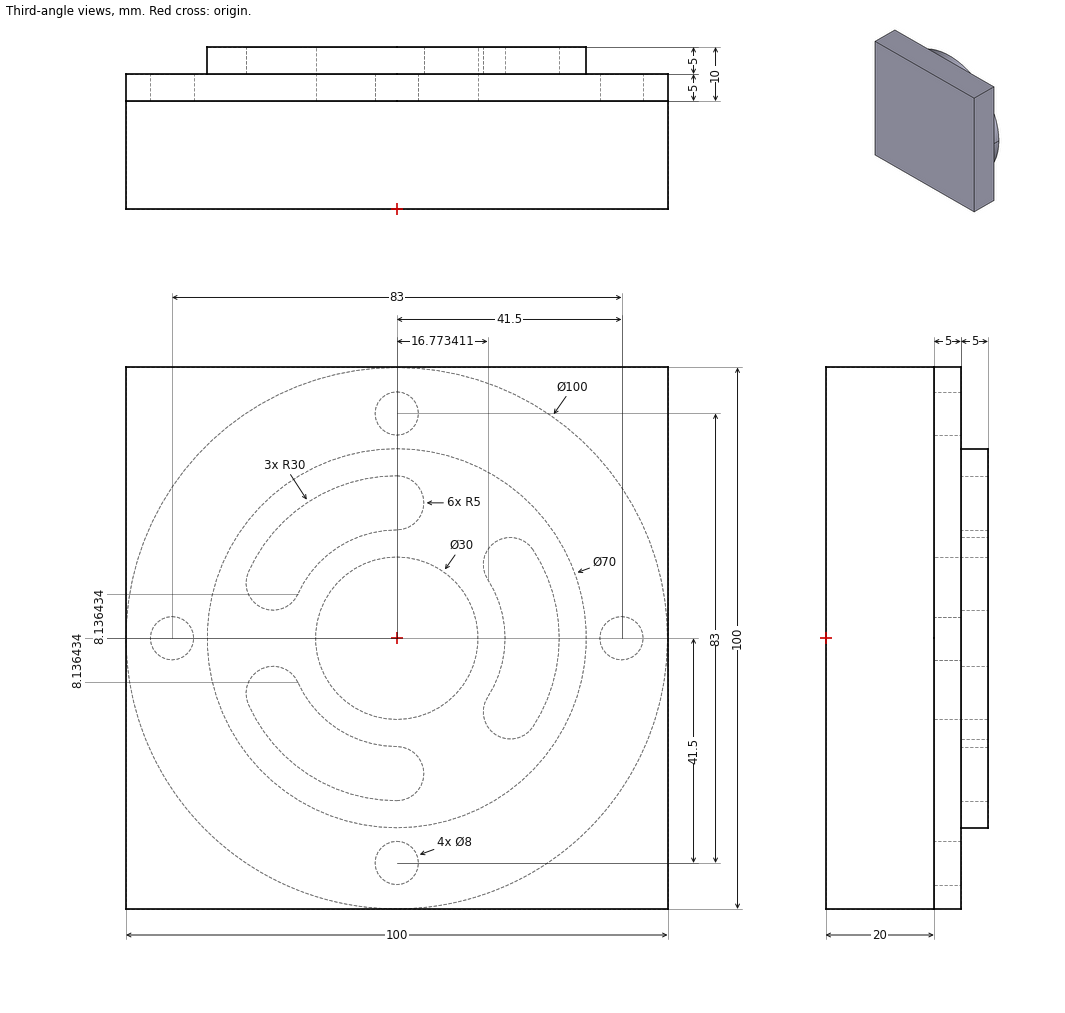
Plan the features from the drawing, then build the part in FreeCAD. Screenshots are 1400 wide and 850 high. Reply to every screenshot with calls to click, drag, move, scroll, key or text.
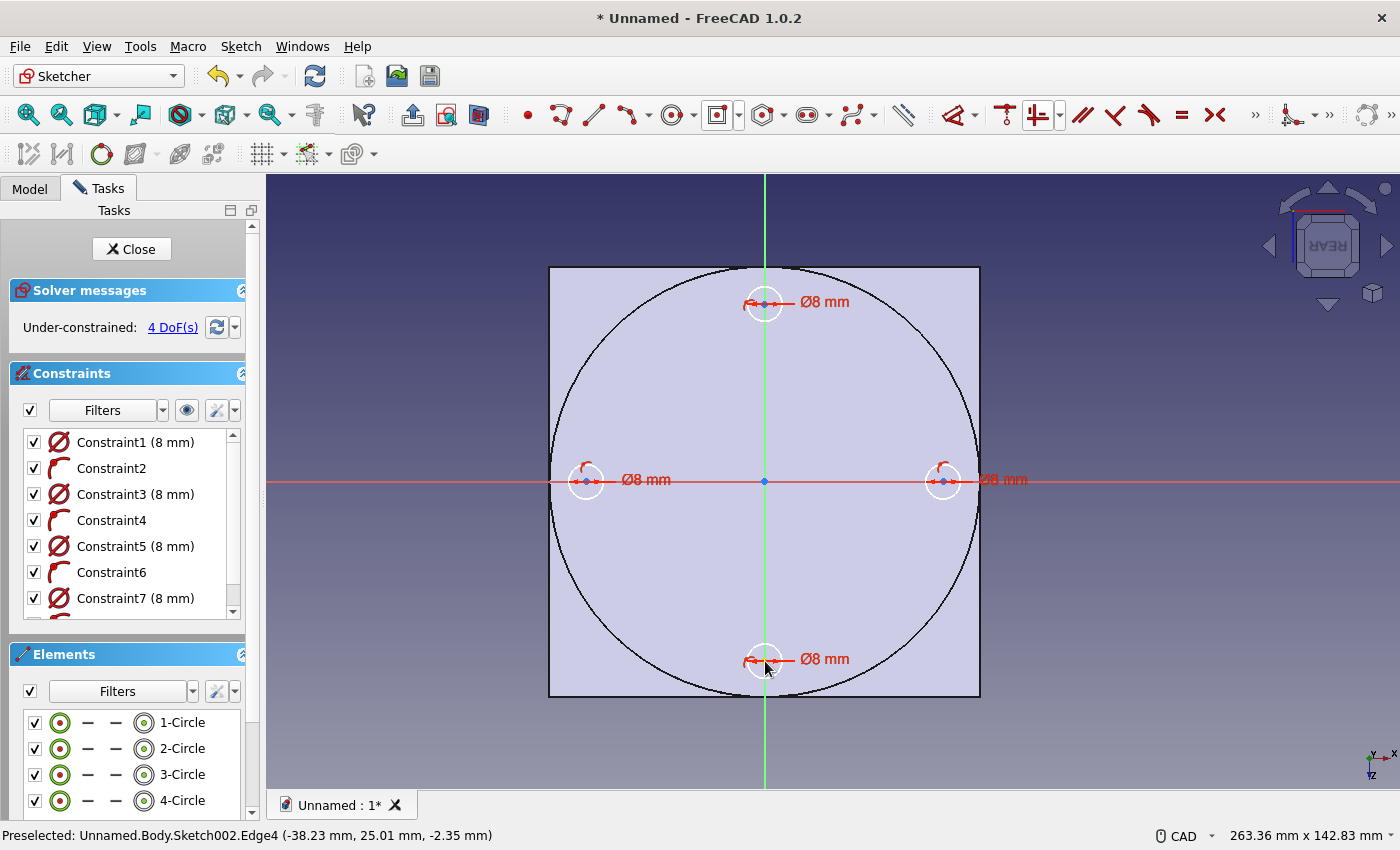
click(765, 304)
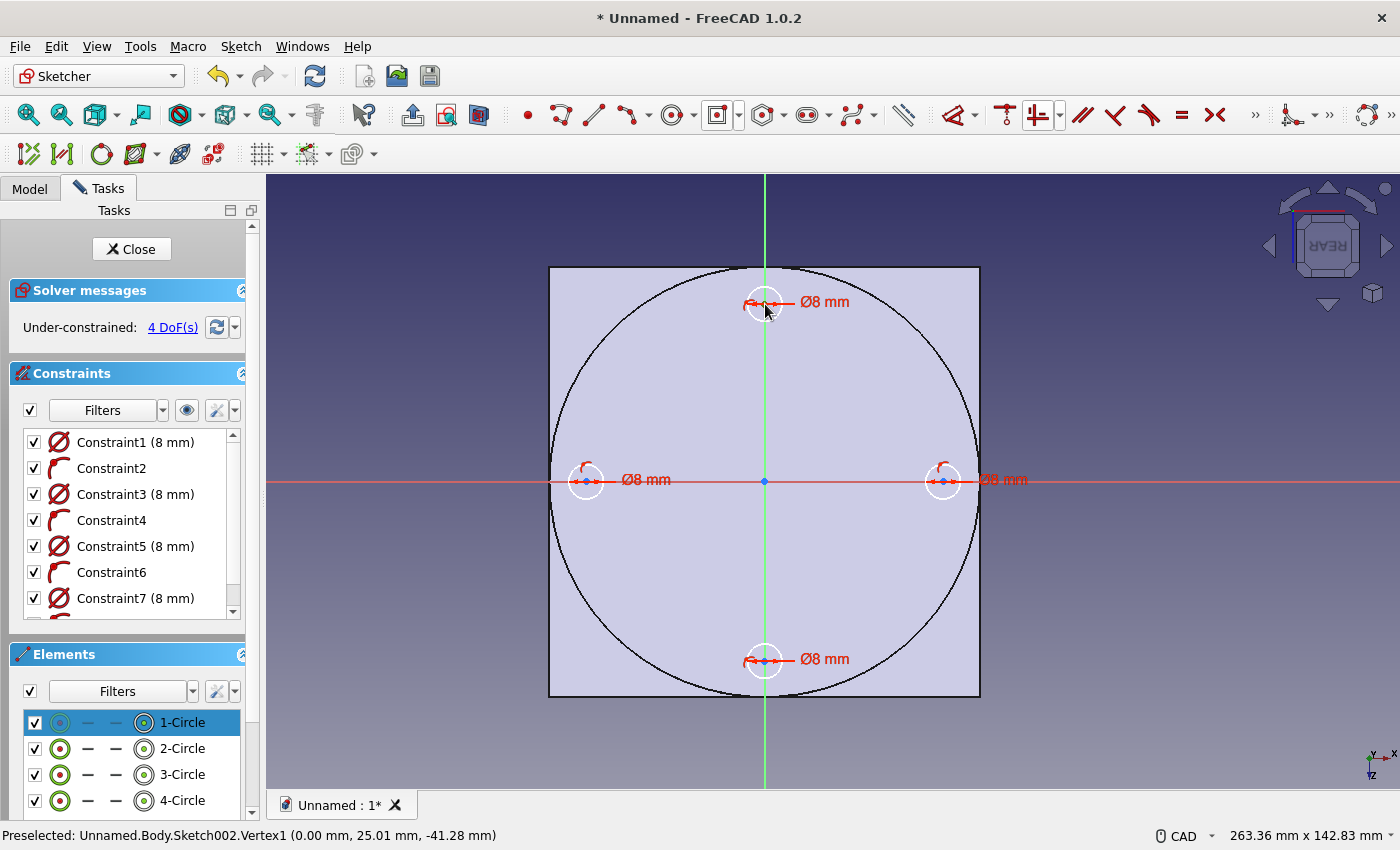
click(765, 661)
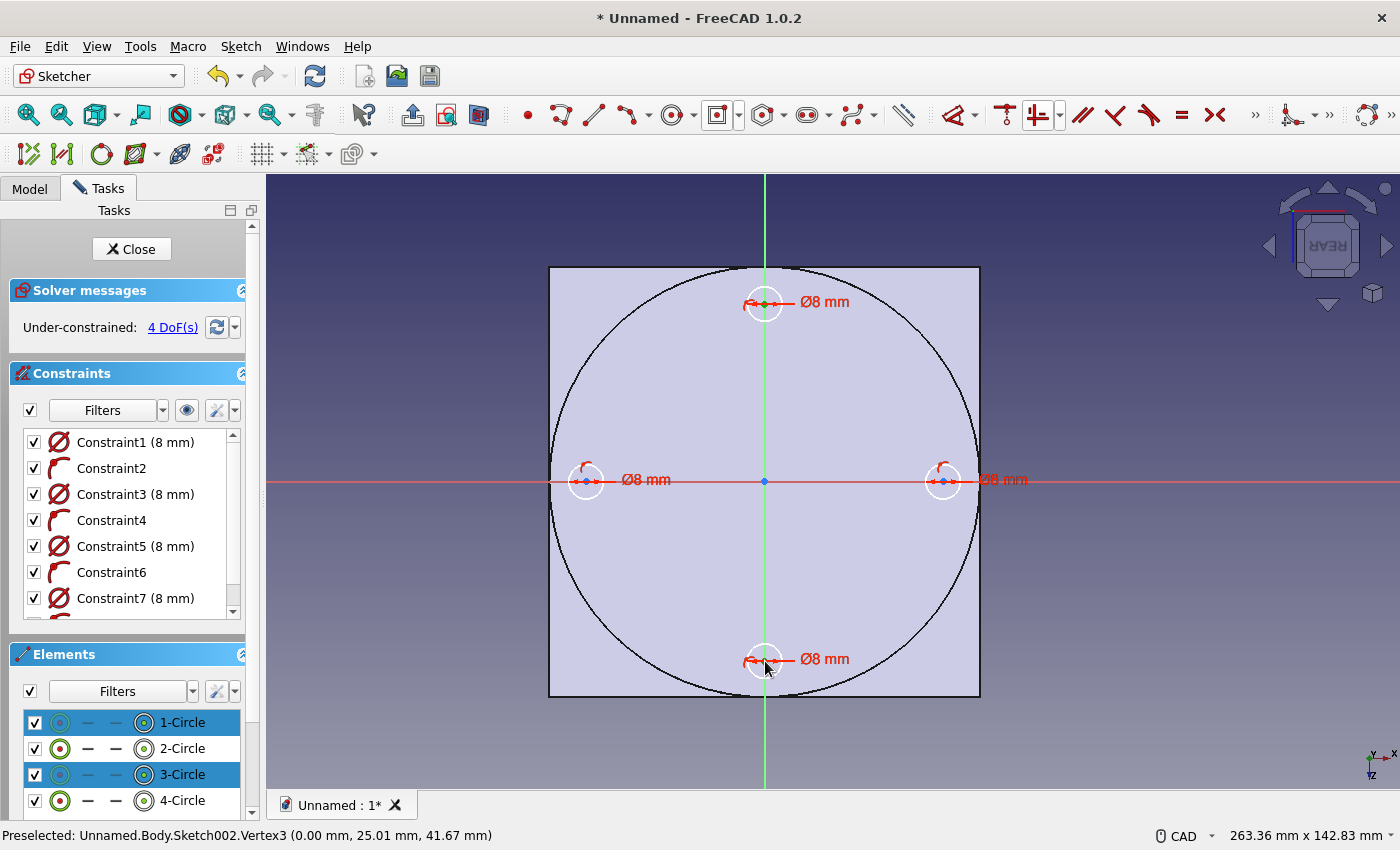
click(974, 116)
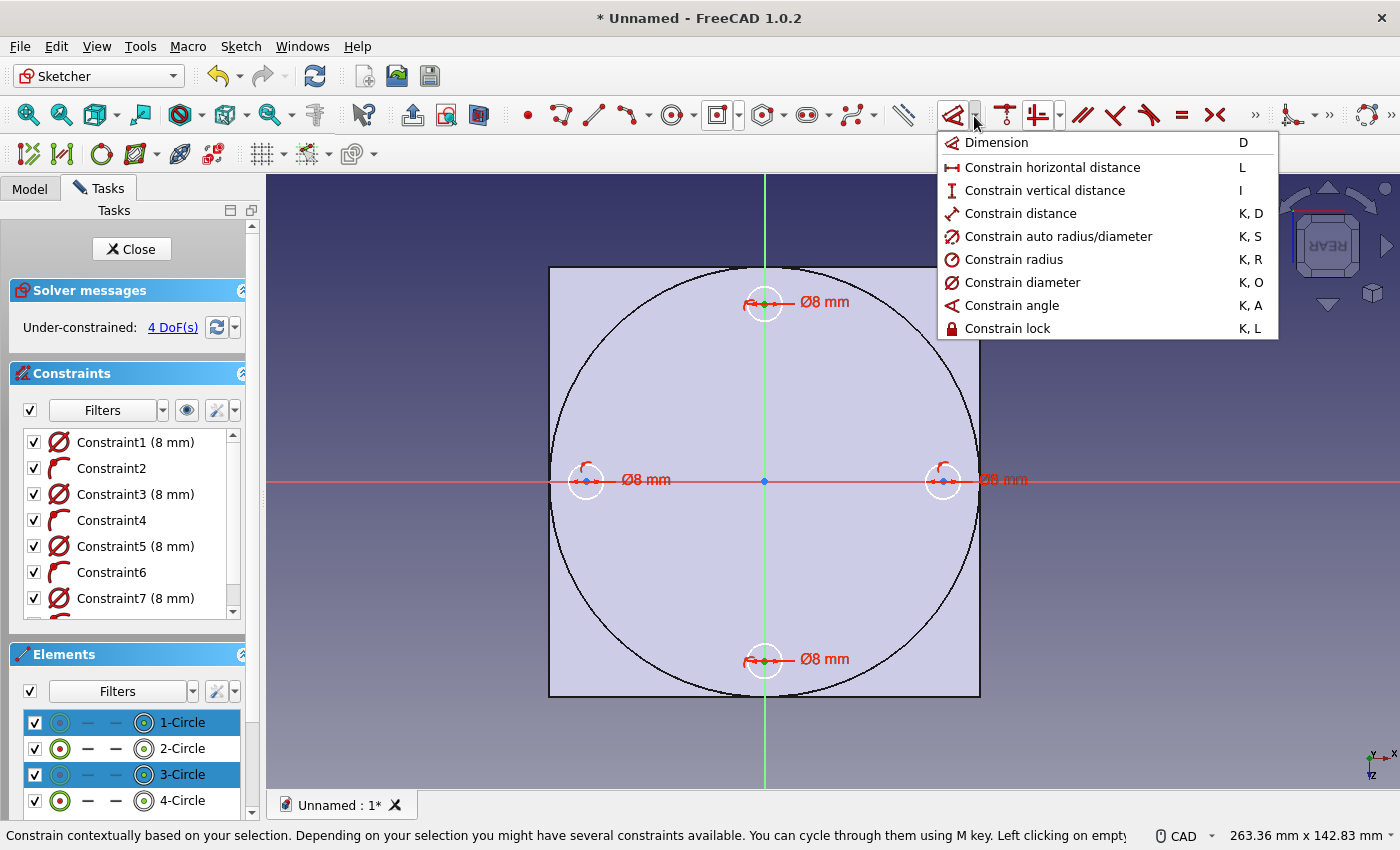
click(1108, 190)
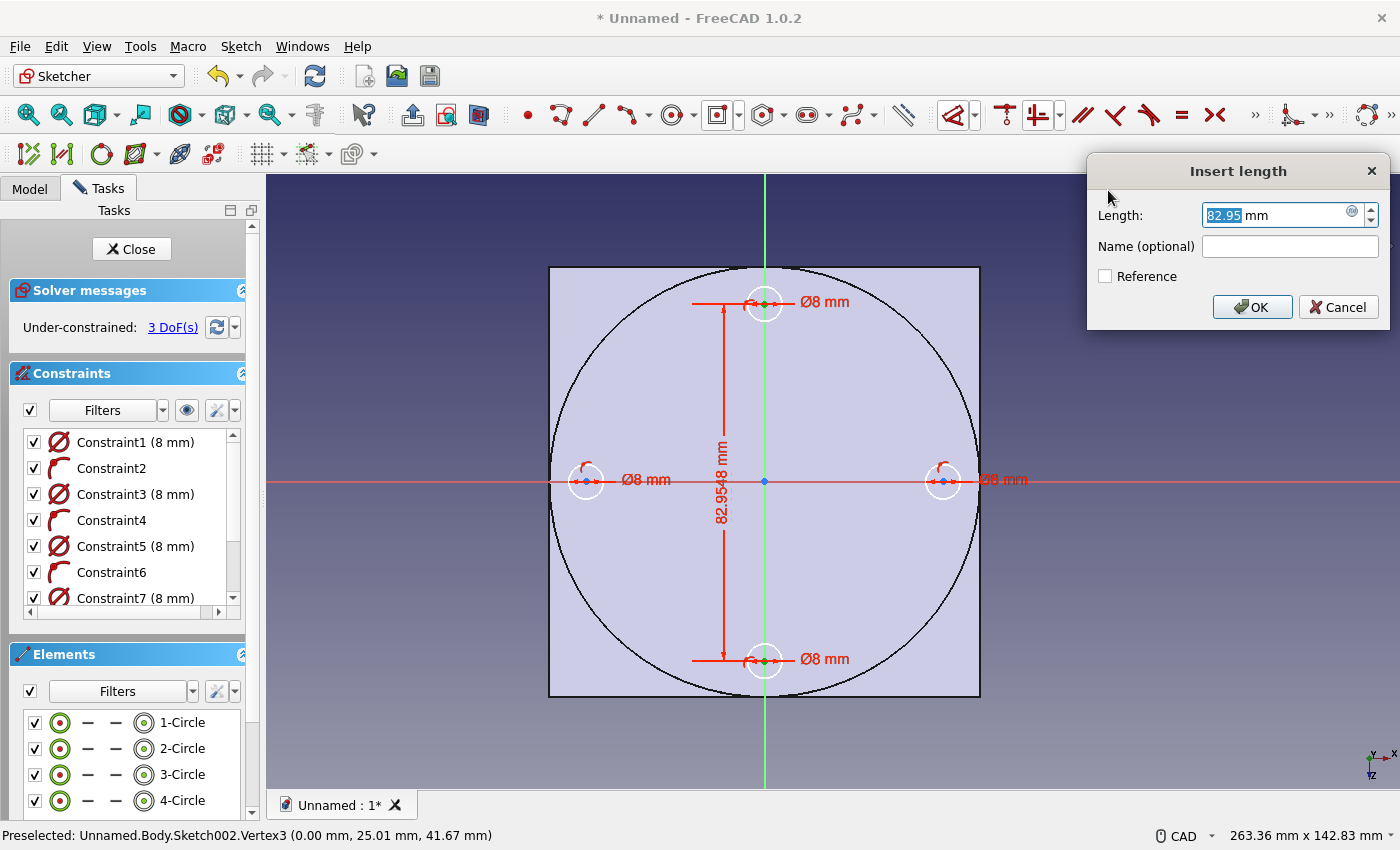
text(83)
key(Return)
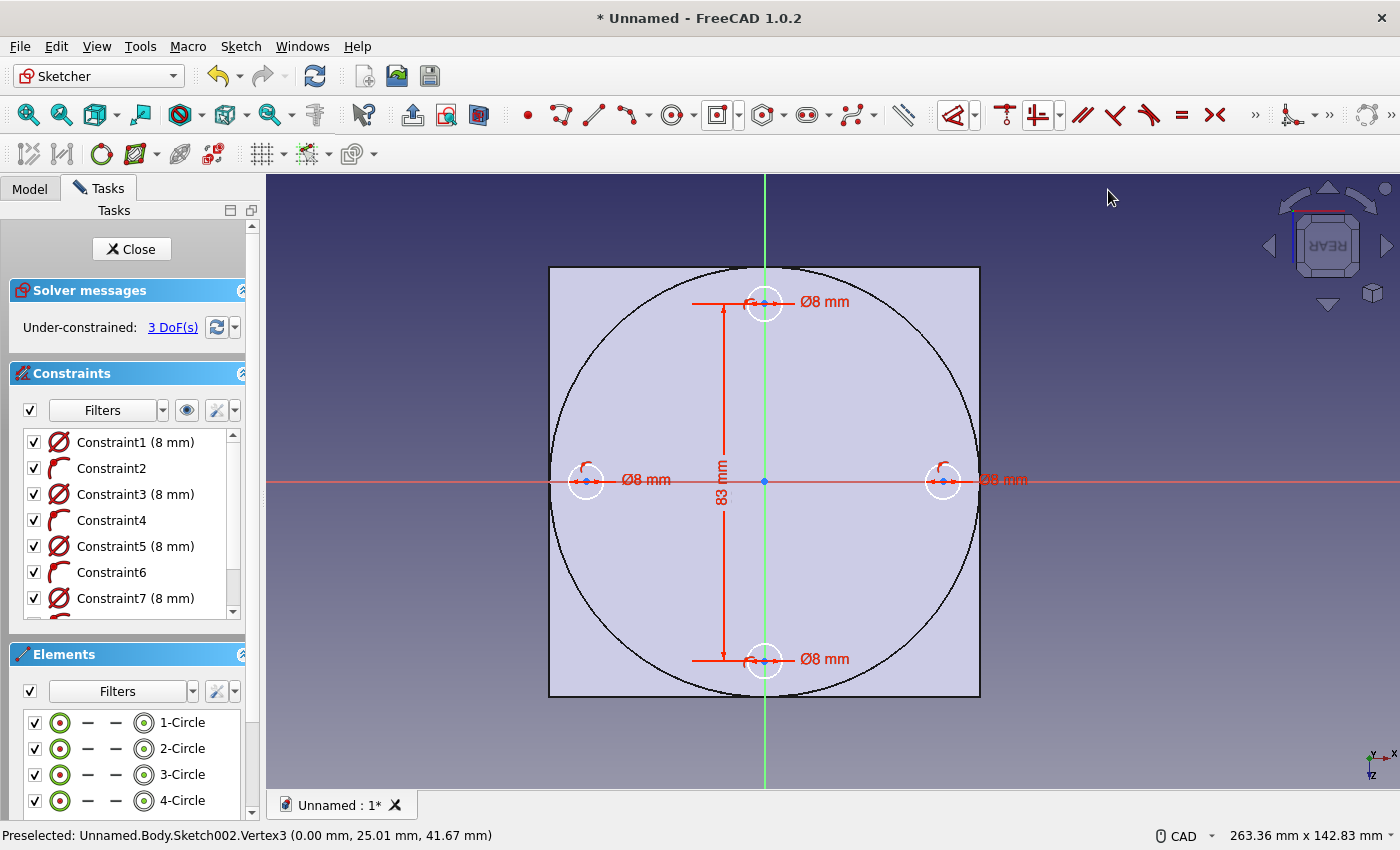
click(943, 482)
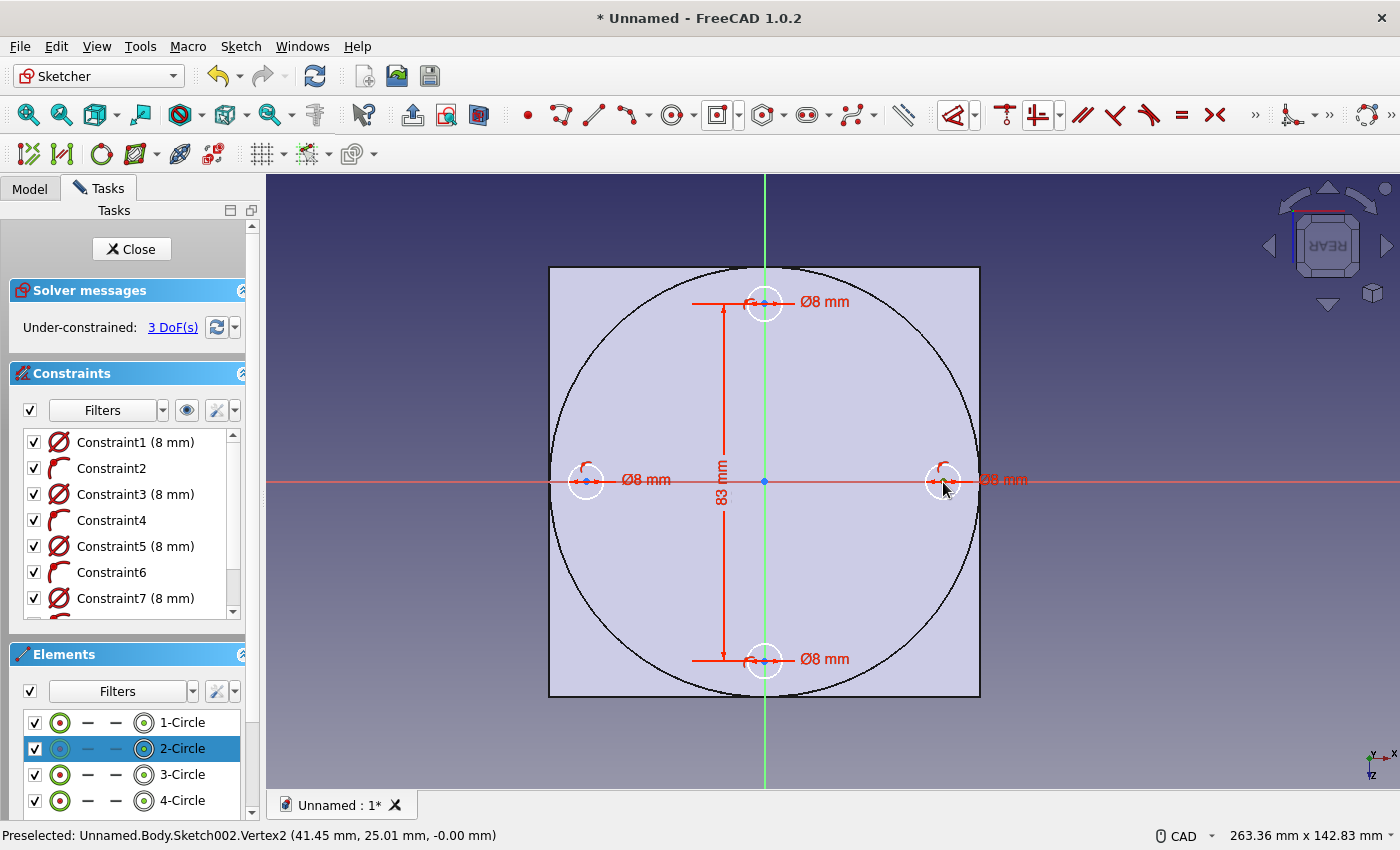
click(586, 482)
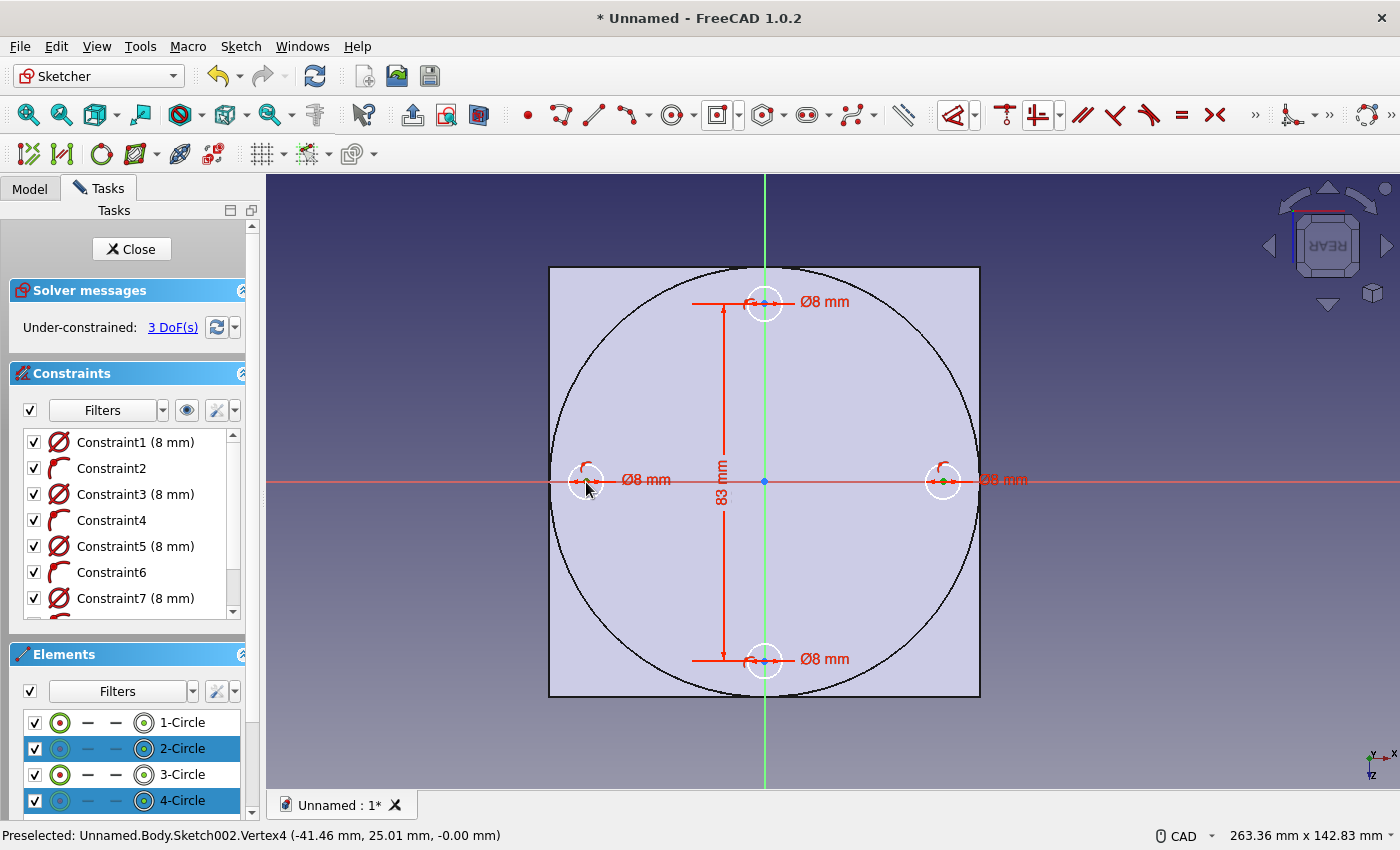
click(974, 116)